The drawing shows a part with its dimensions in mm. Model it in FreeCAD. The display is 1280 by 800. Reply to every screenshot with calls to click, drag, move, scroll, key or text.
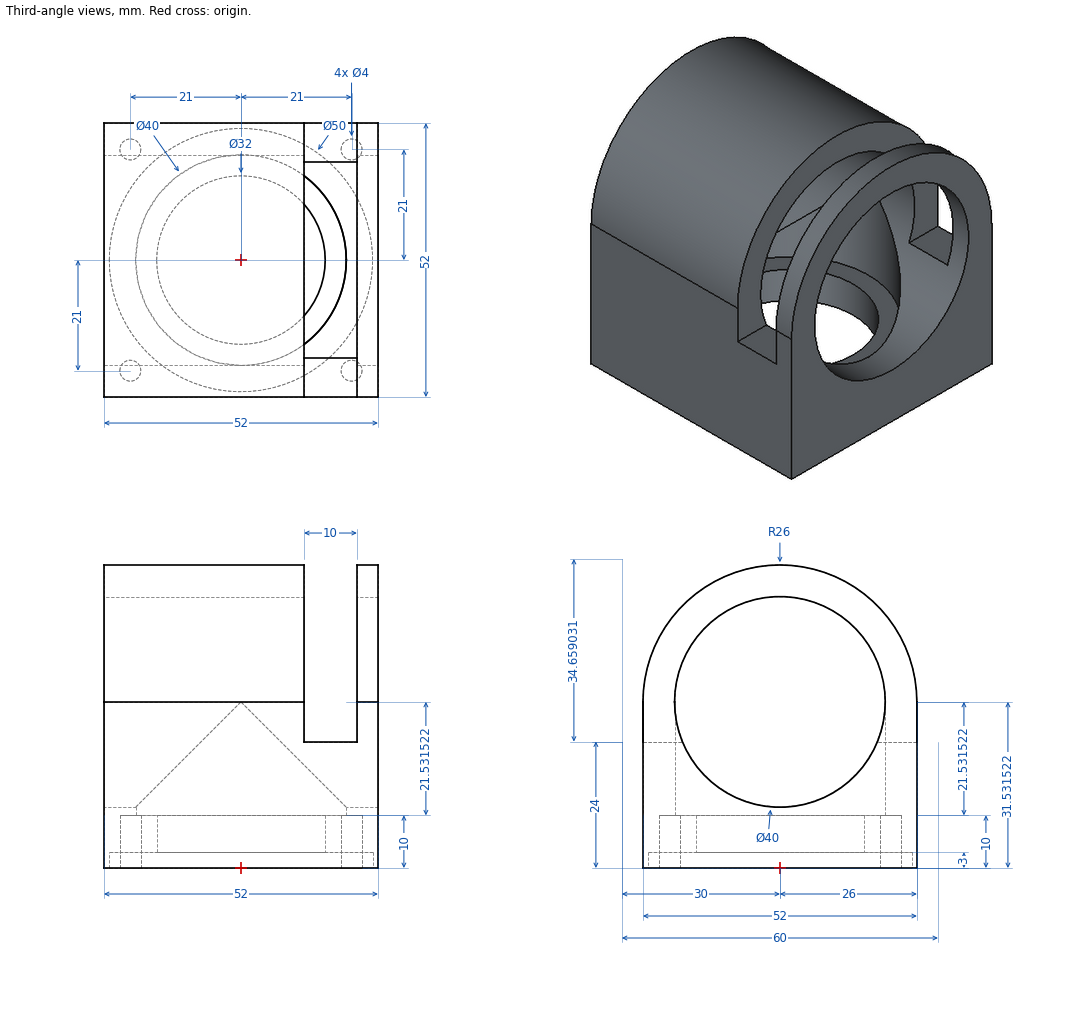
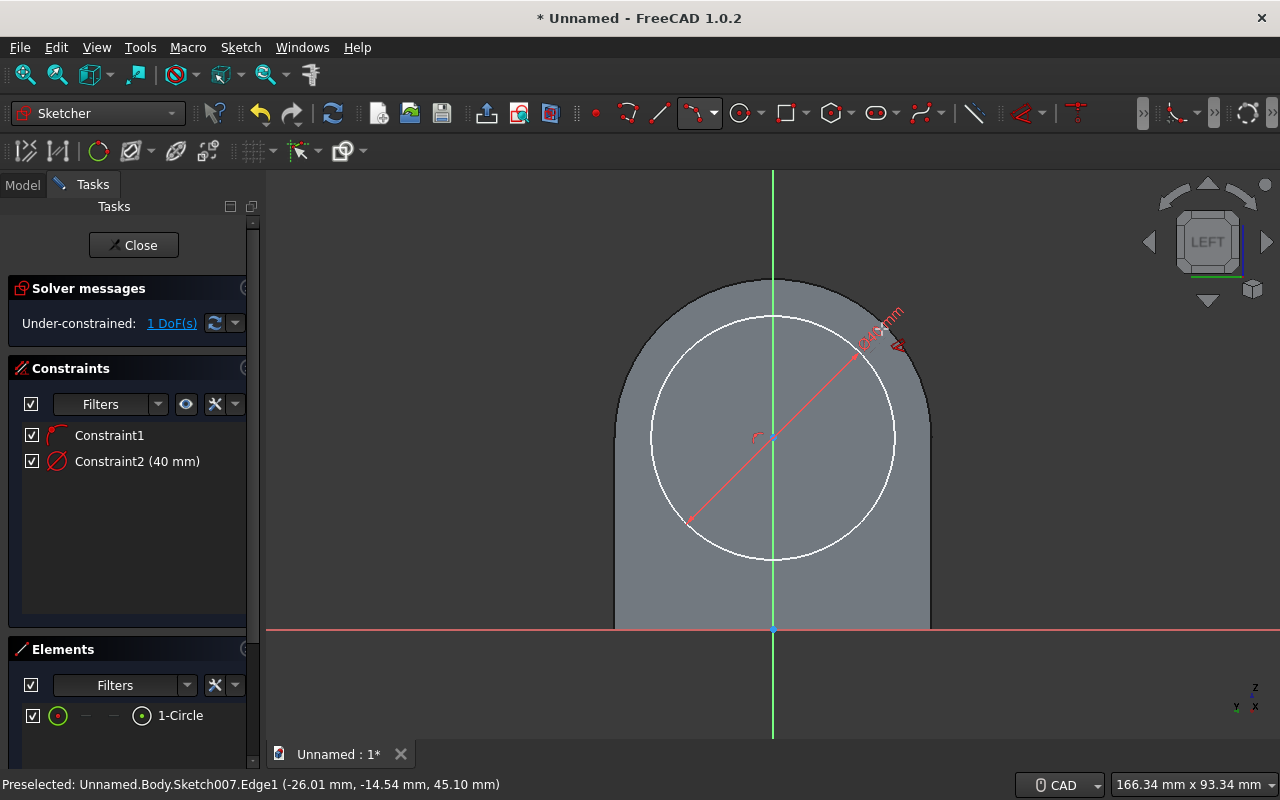
click(773, 438)
click(807, 534)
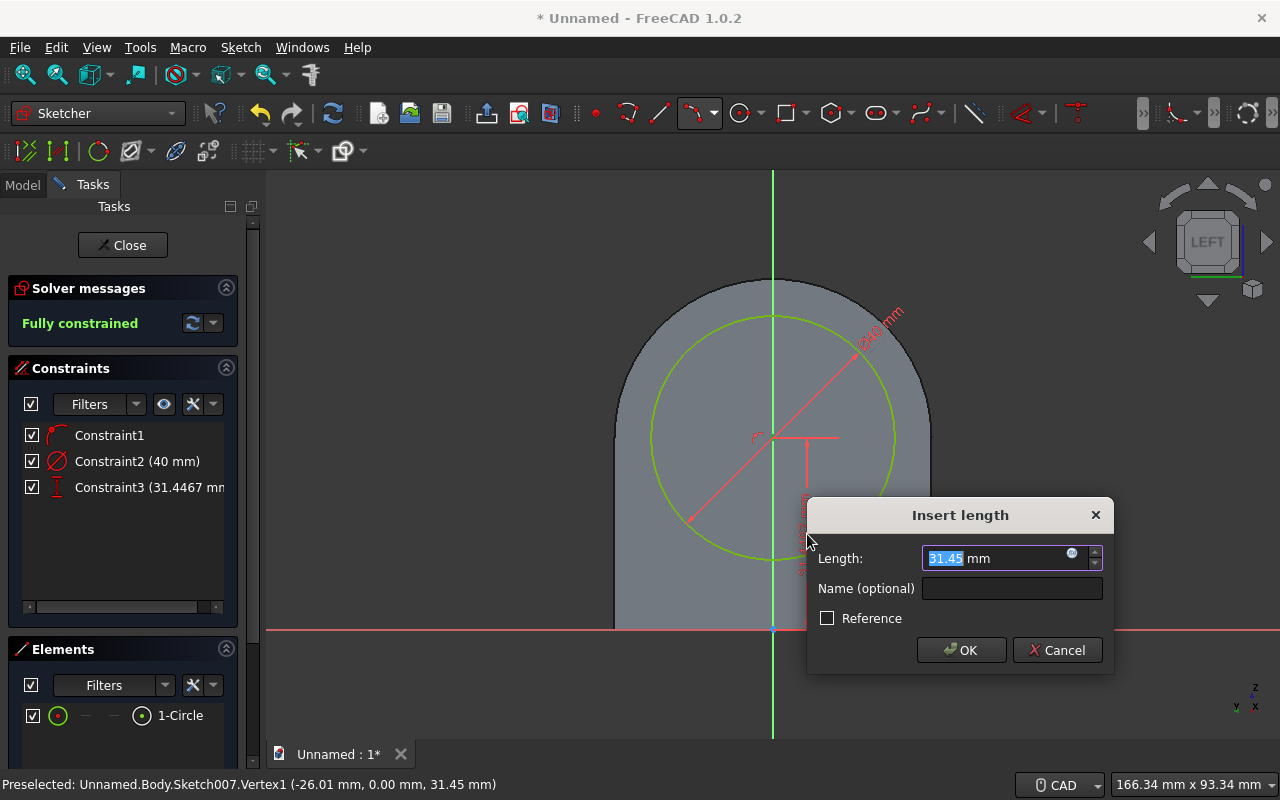
text(31.531522)
key(Return)
key(Escape)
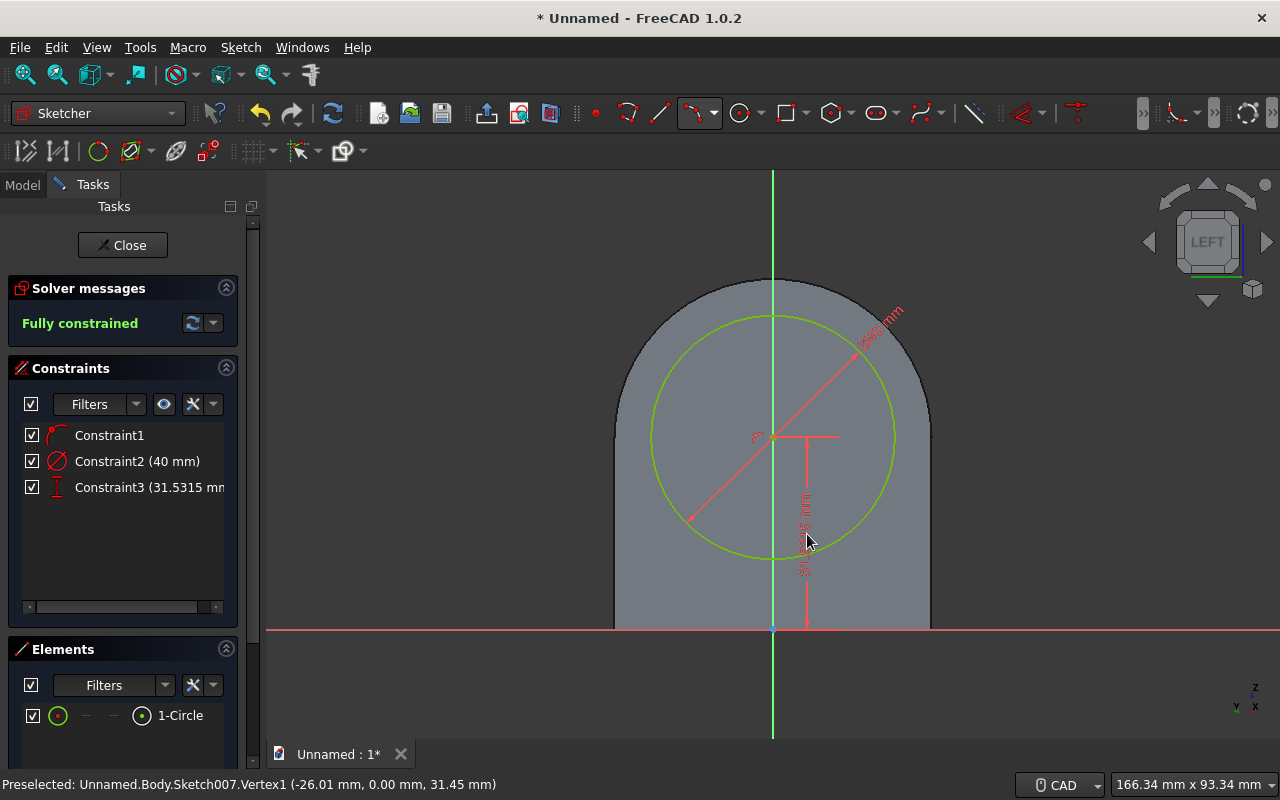
click(123, 245)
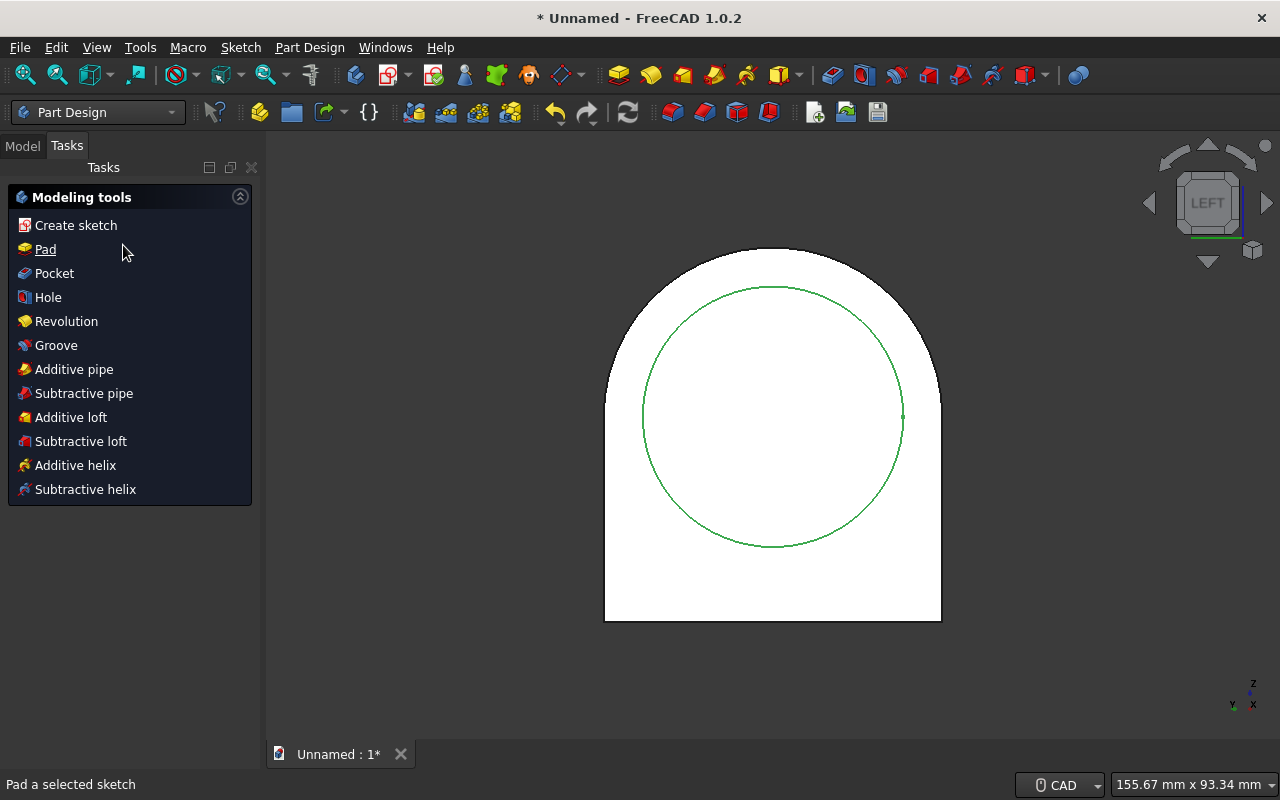
click(834, 76)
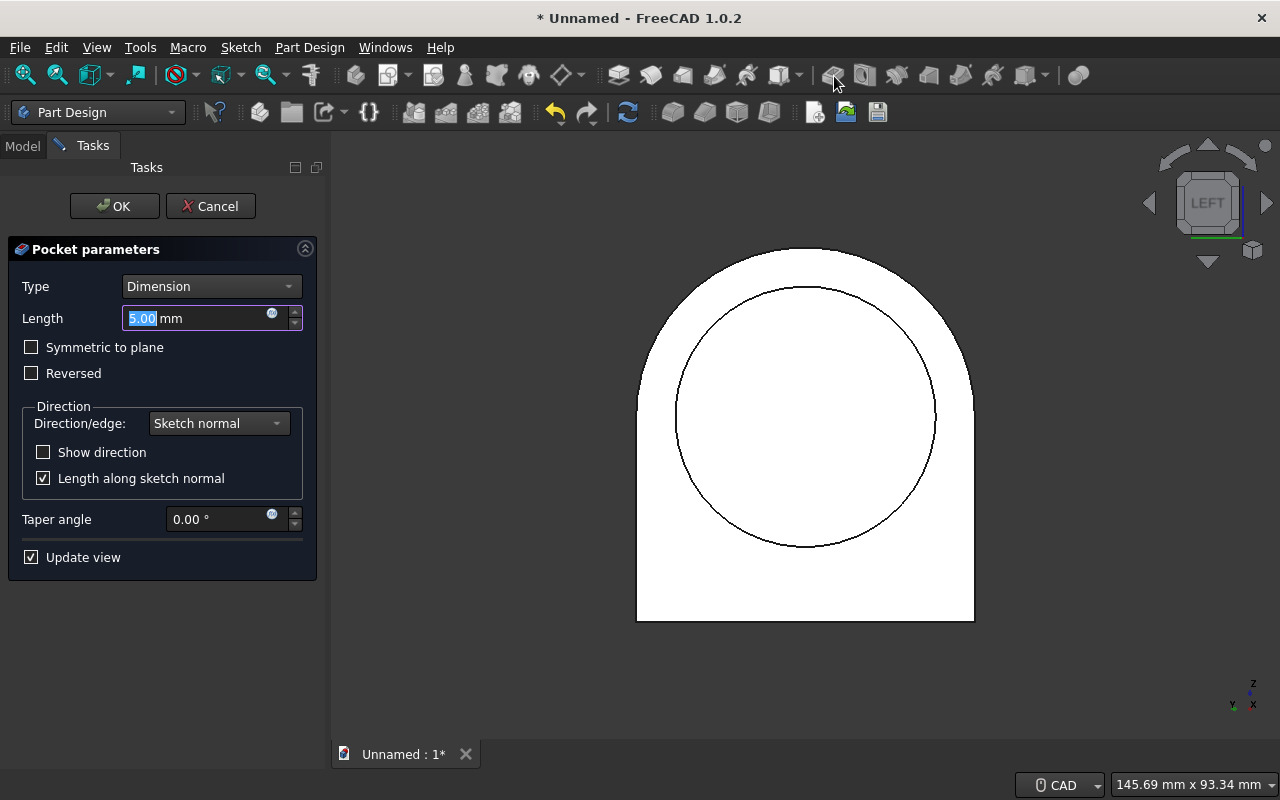
text(52)
key(Tab)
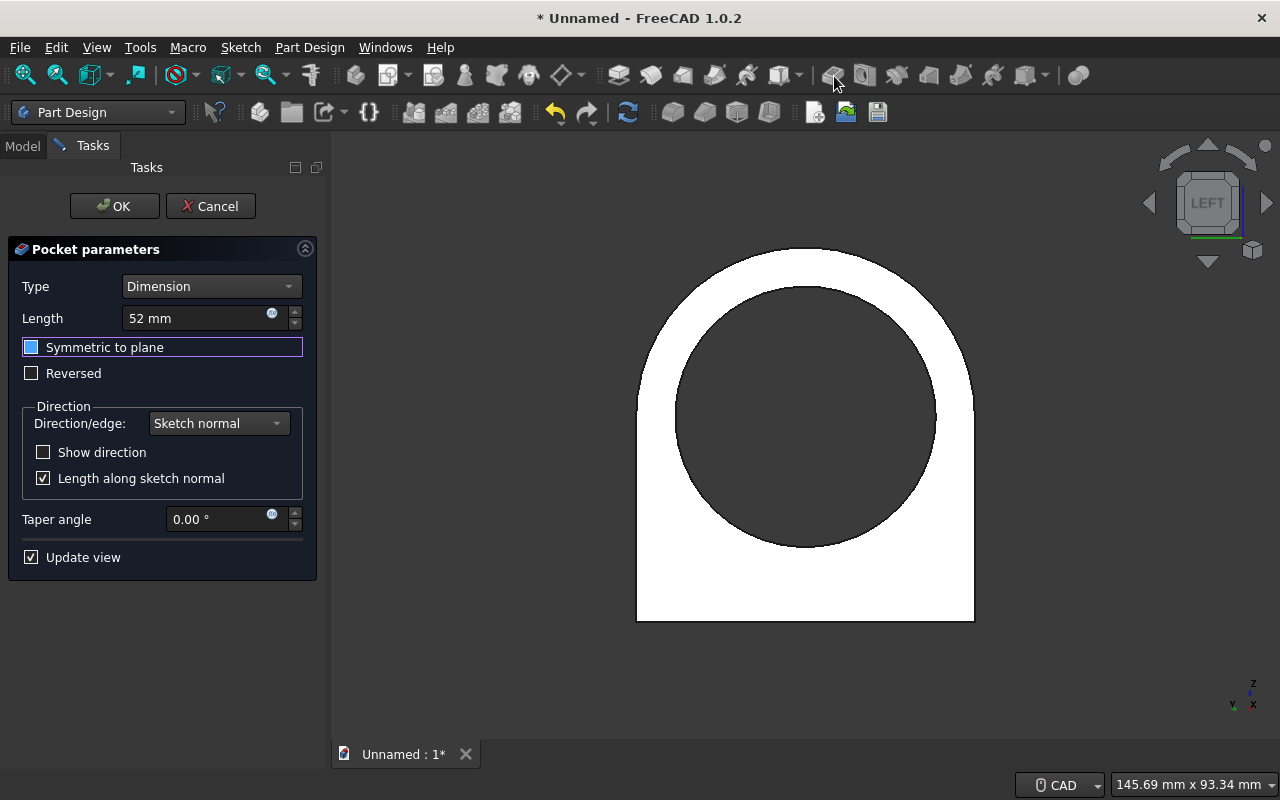
click(115, 206)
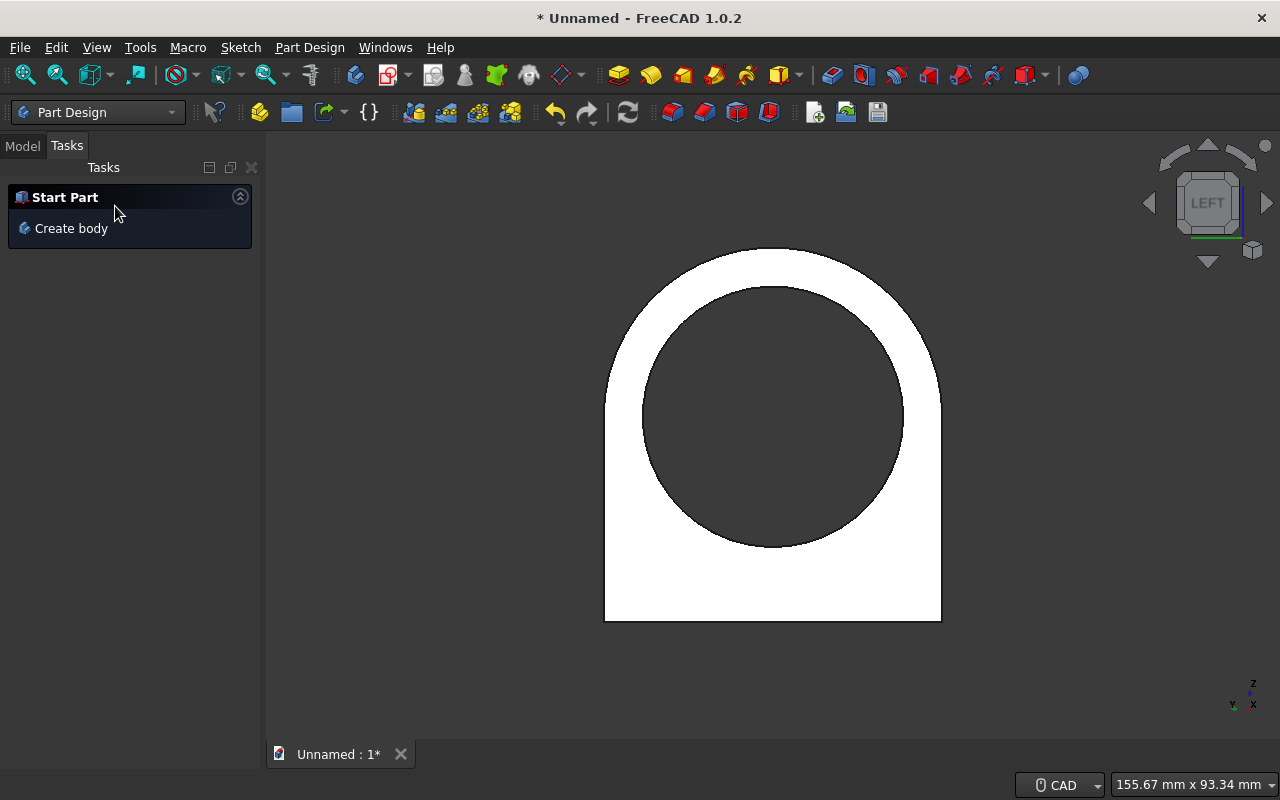
click(23, 145)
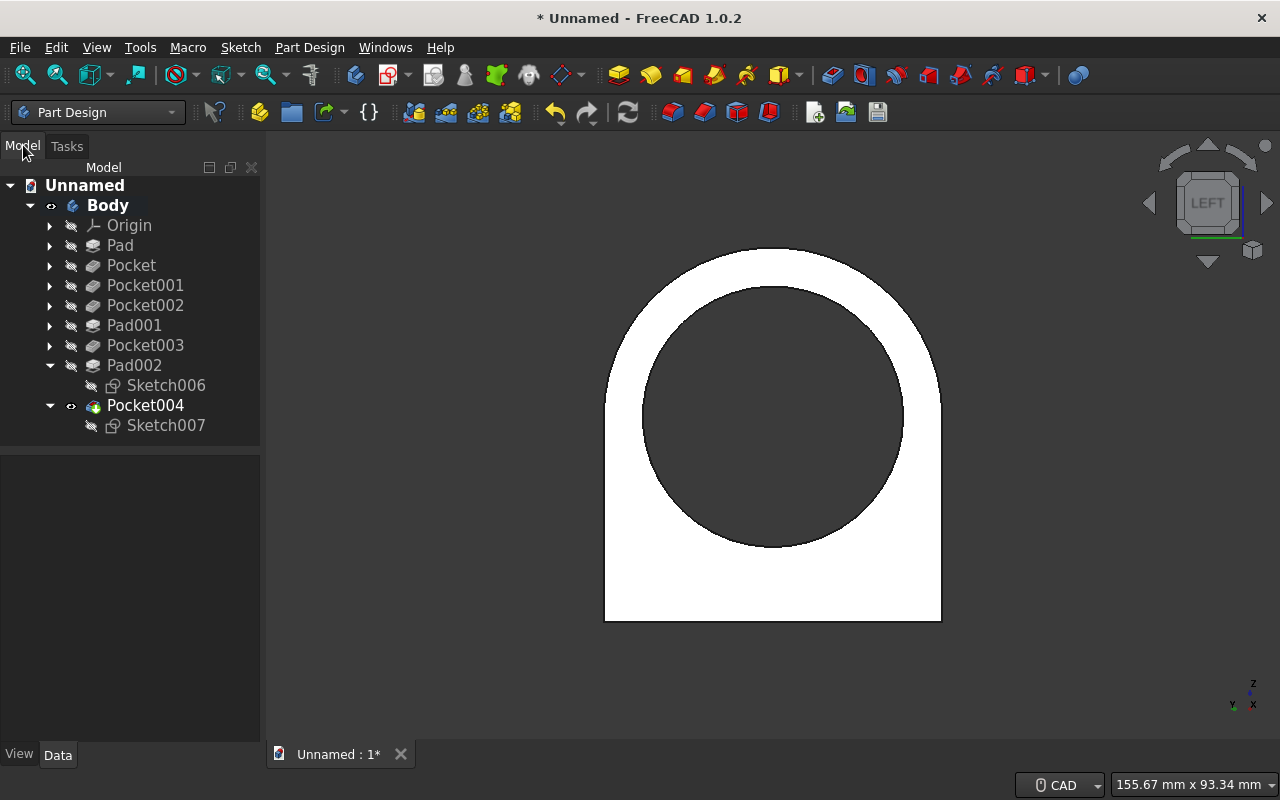
click(50, 226)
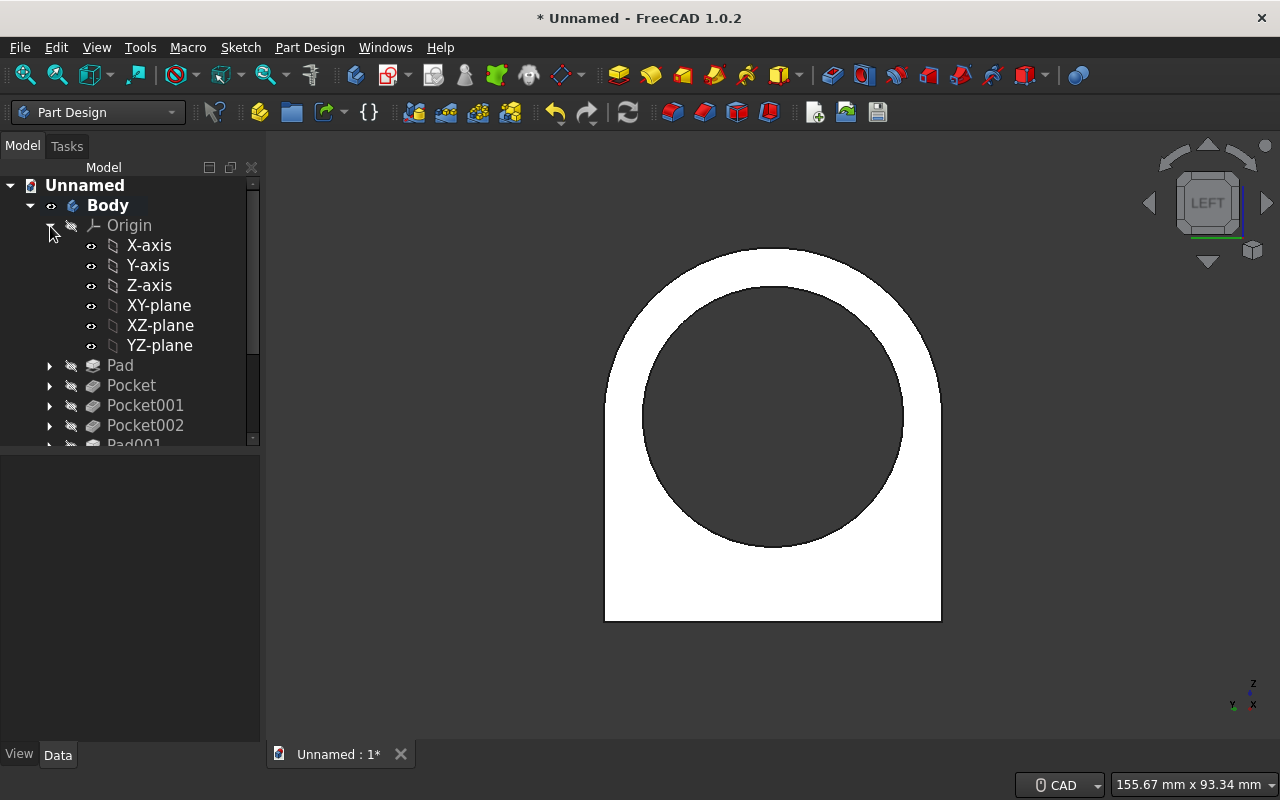
click(136, 346)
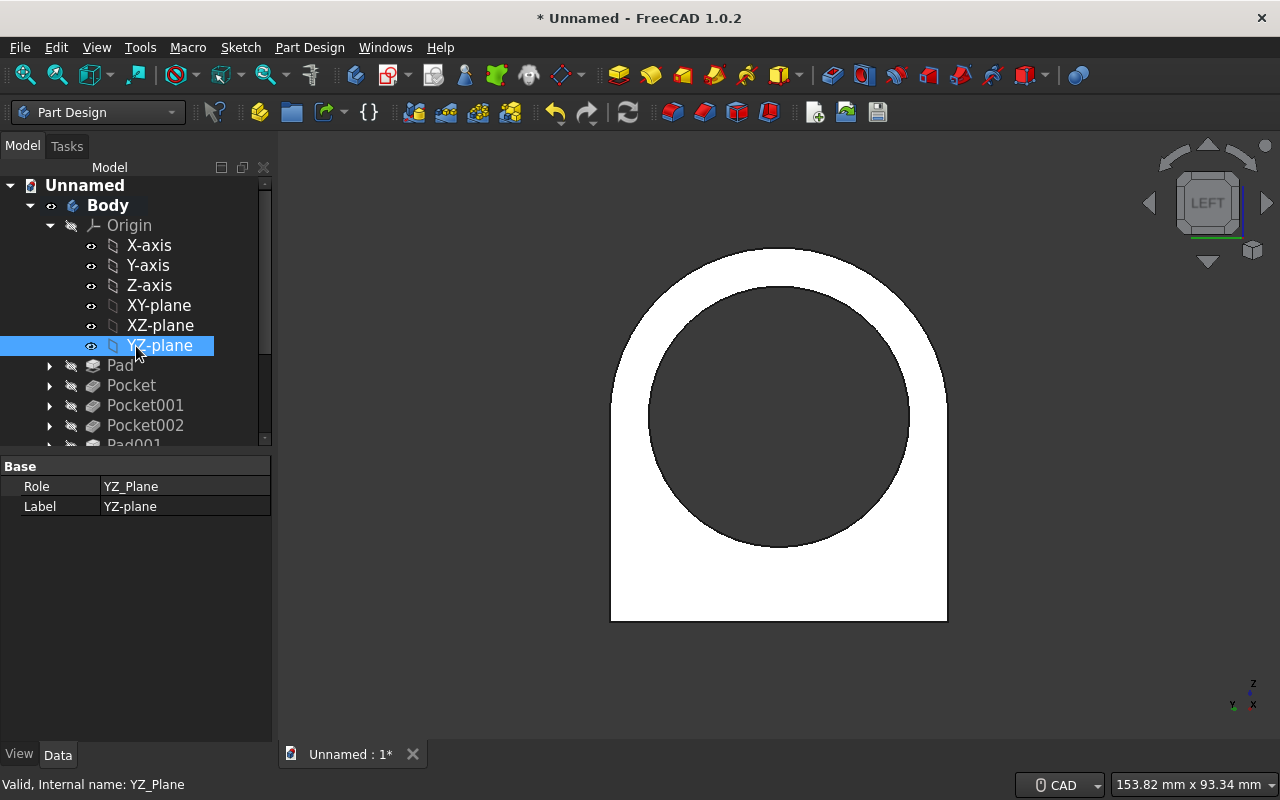
click(562, 76)